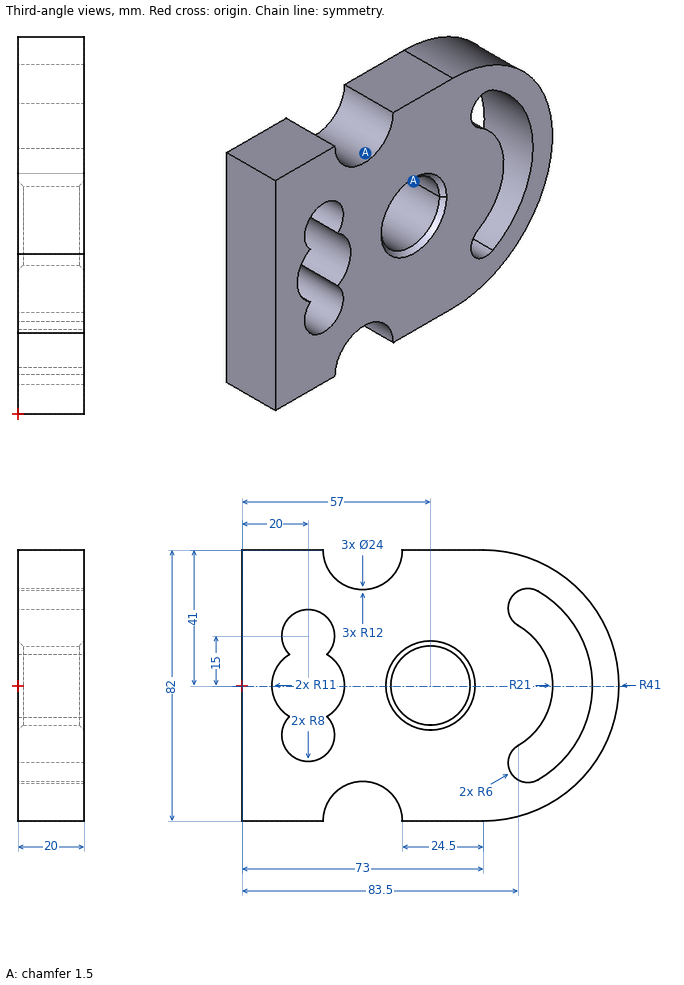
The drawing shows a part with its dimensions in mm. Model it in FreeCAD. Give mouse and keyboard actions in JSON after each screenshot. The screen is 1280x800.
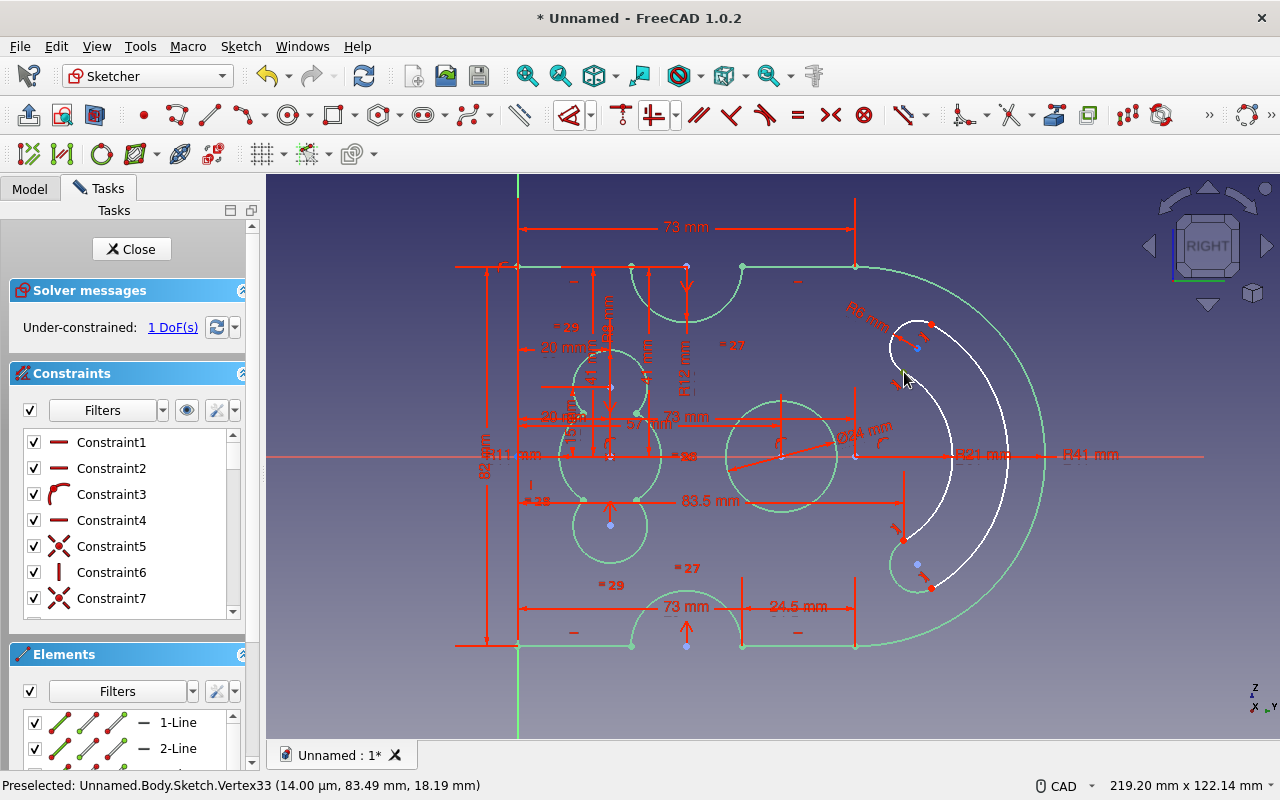
{"action": "key", "text": "l"}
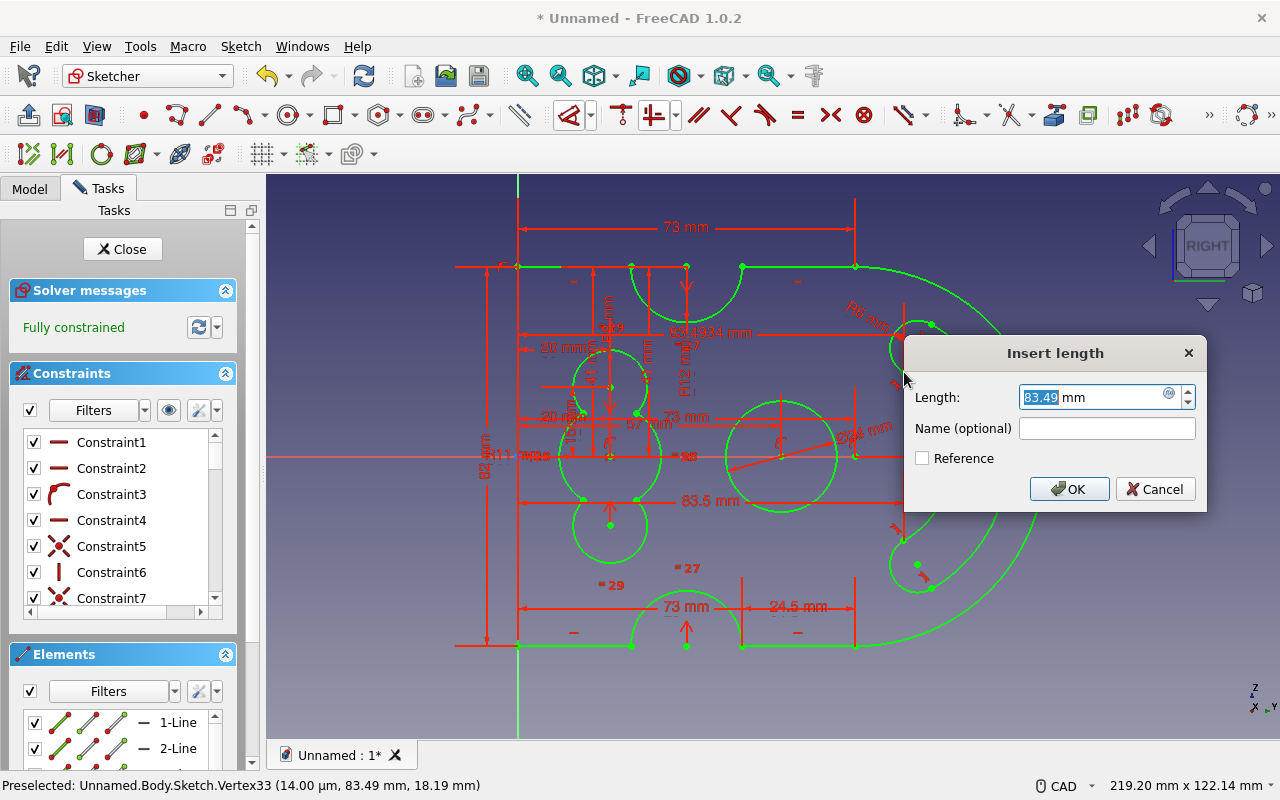
{"action": "type", "text": "83.5"}
{"action": "key", "text": "Return"}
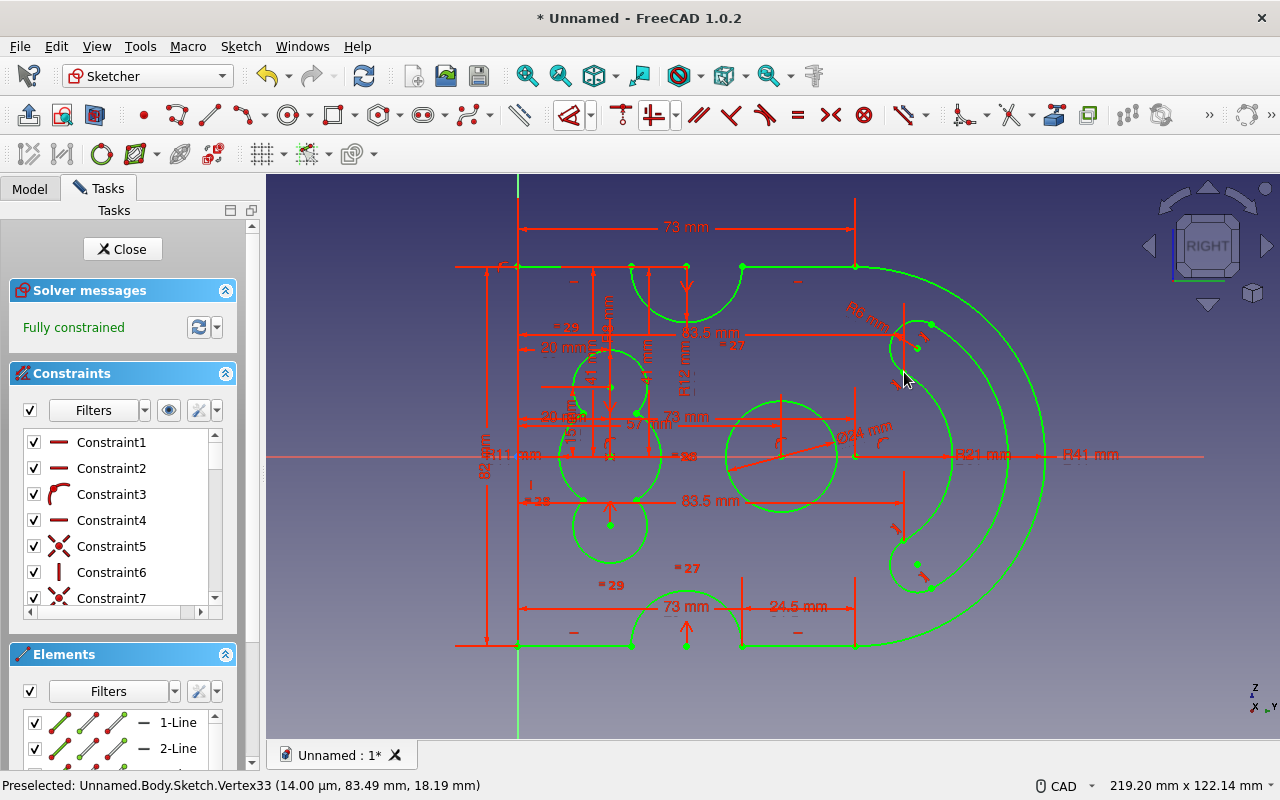
{"action": "left_click", "coordinate": [123, 249]}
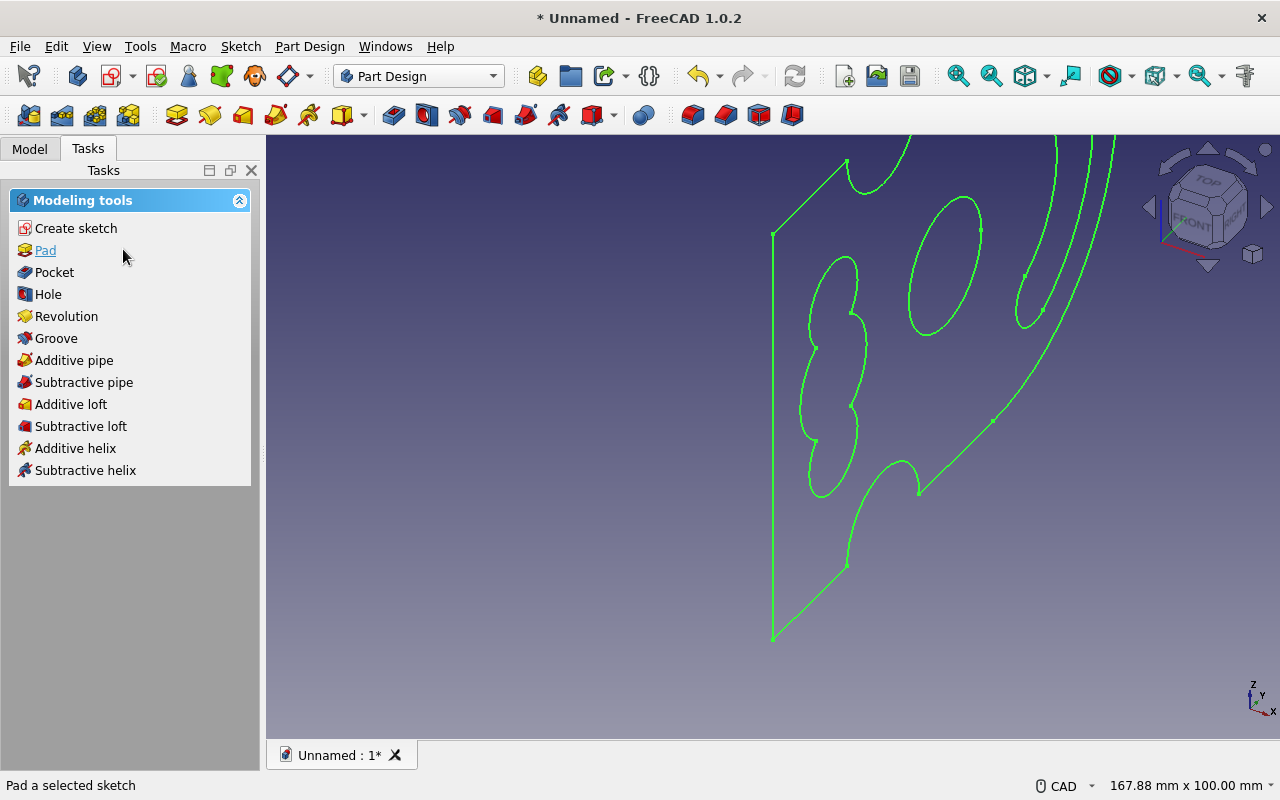
{"action": "left_click", "coordinate": [177, 116]}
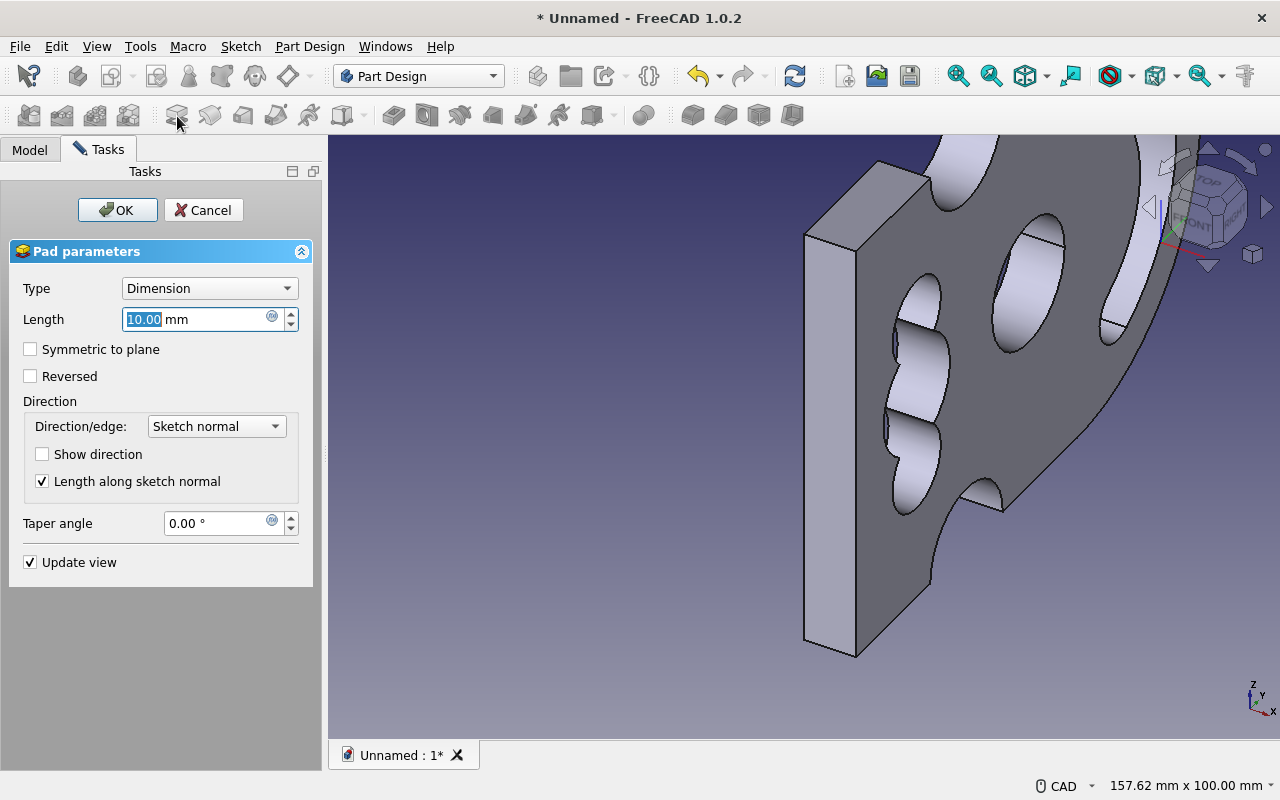
{"action": "type", "text": "20"}
{"action": "key", "text": "Tab"}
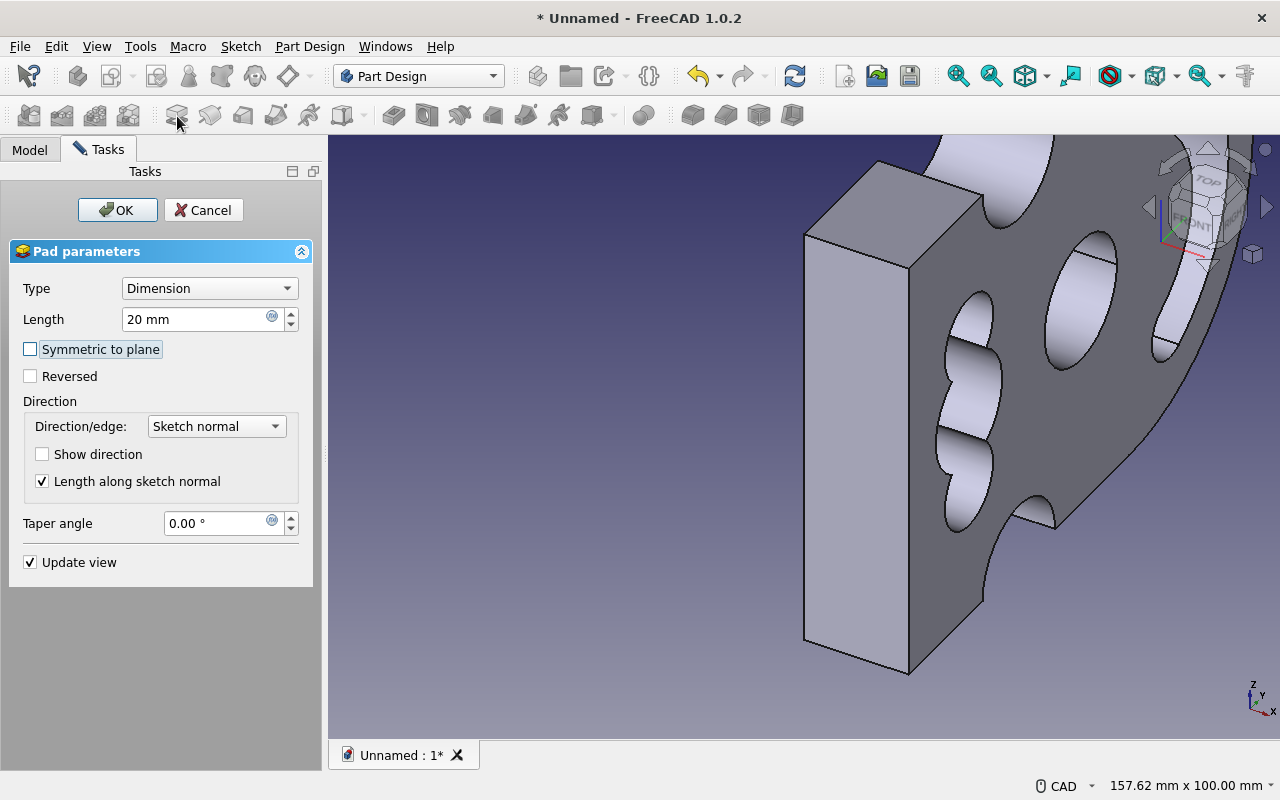
{"action": "left_click", "coordinate": [118, 210]}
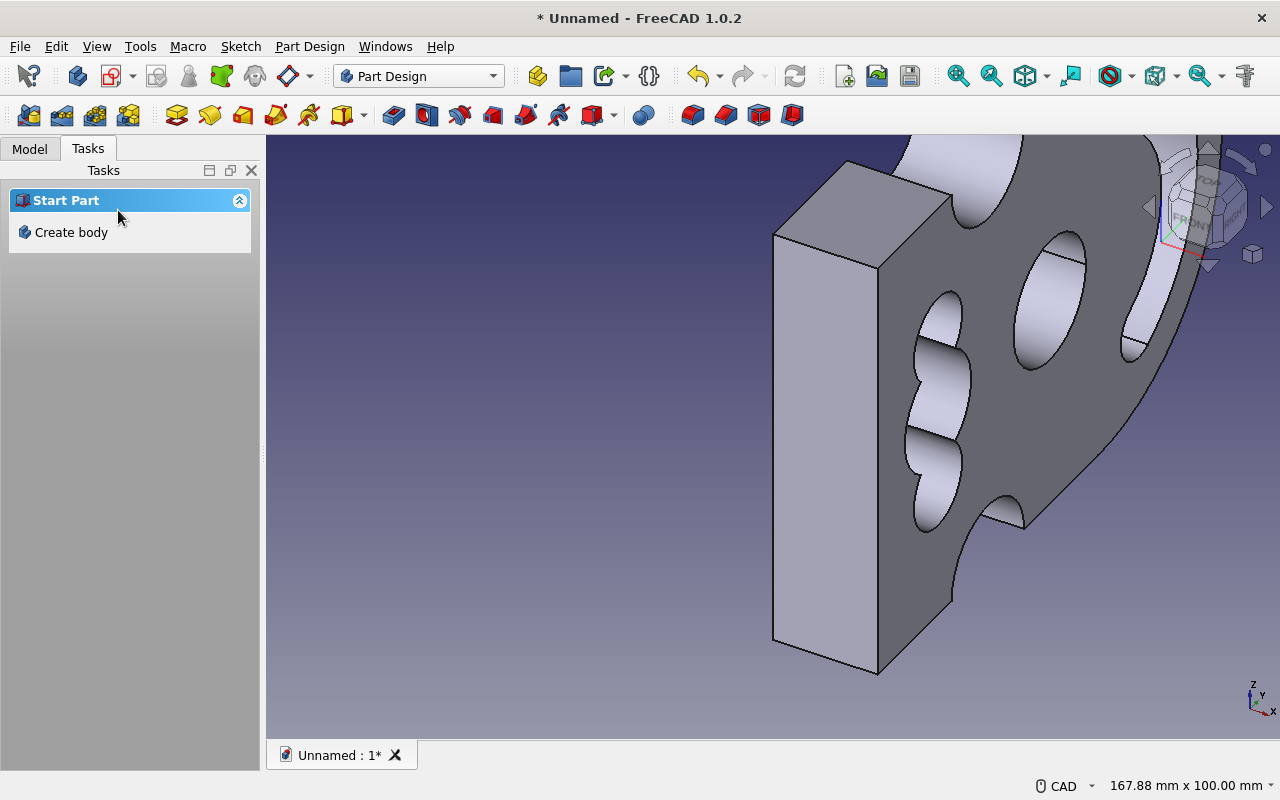
{"action": "left_click", "coordinate": [959, 76]}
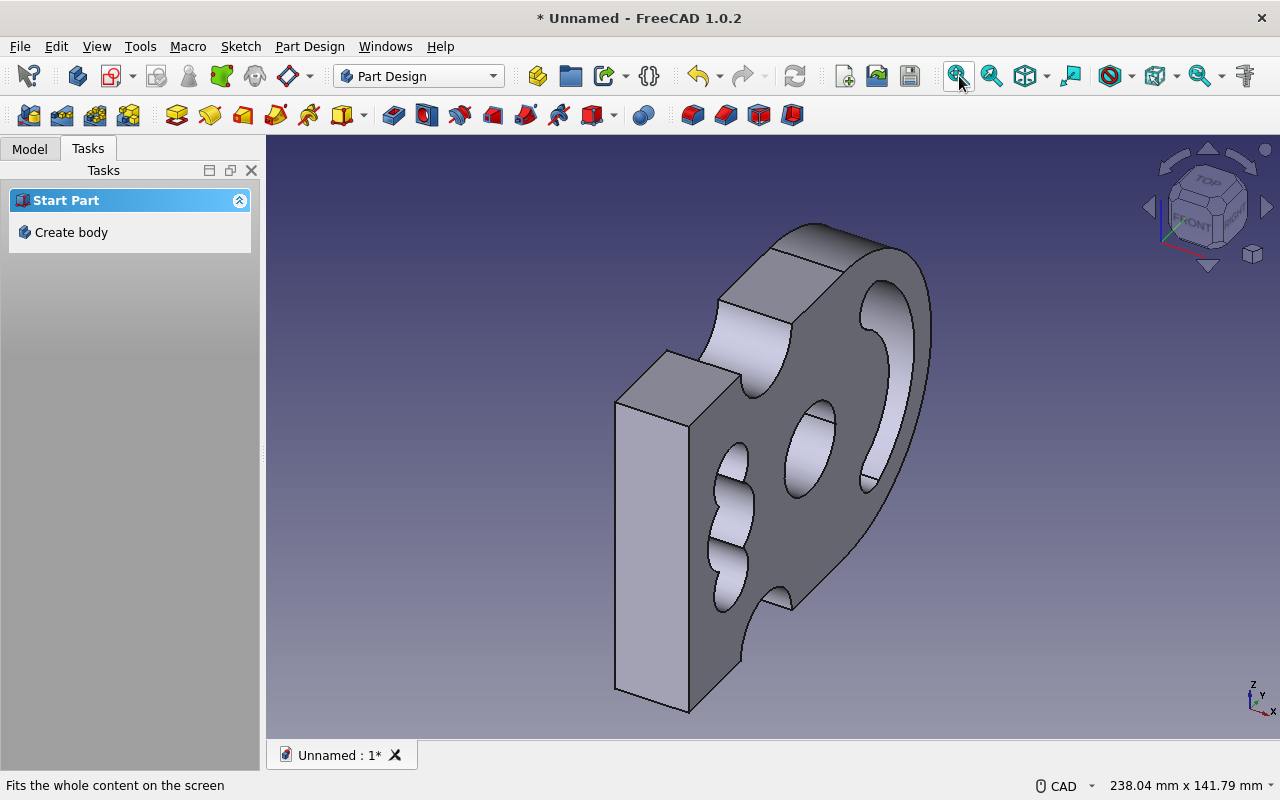
{"action": "left_click", "coordinate": [802, 496]}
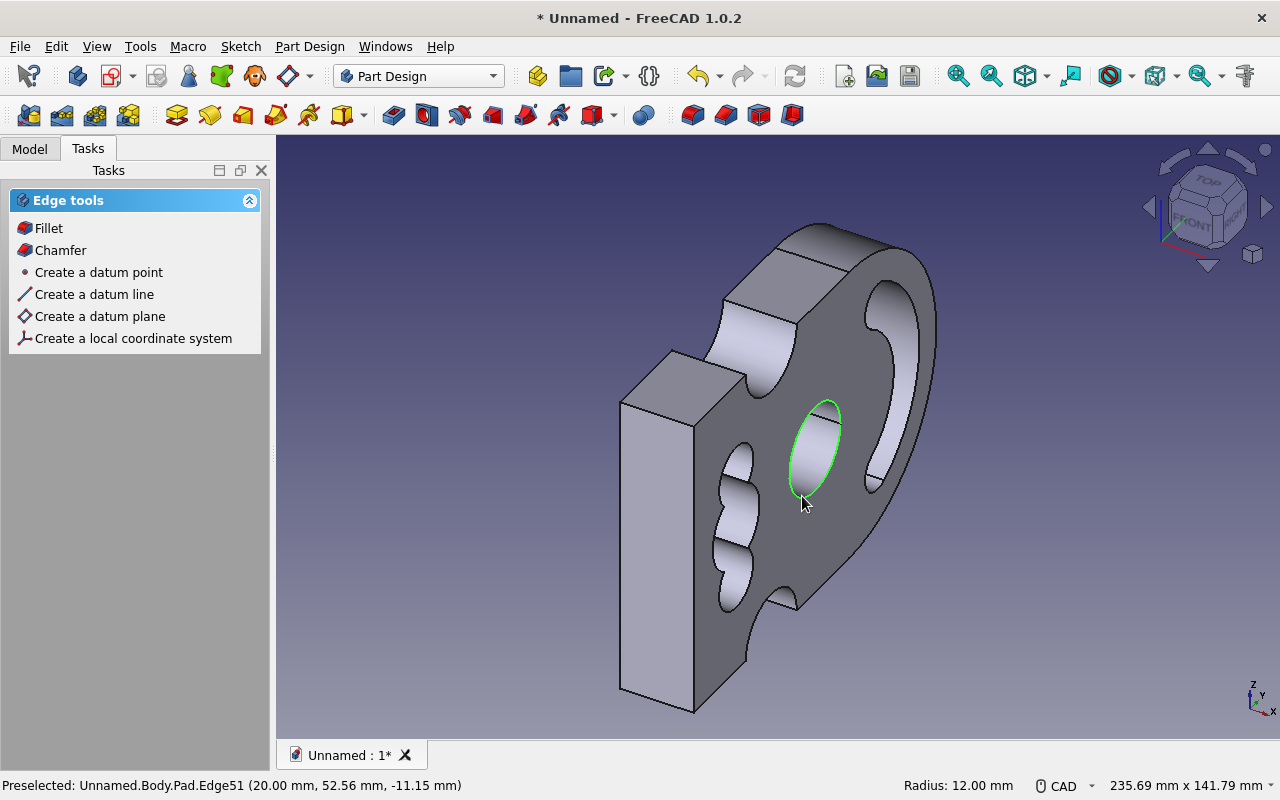
{"action": "key", "text": "0"}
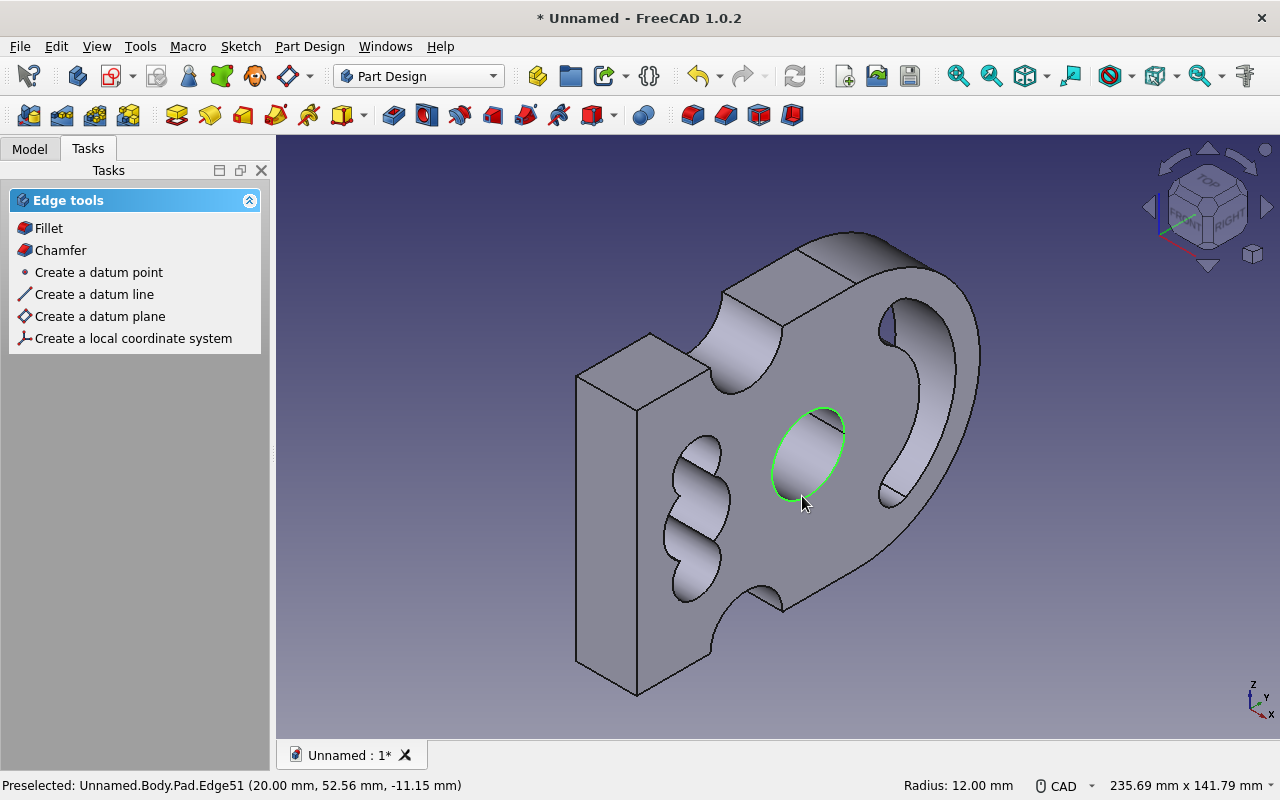
{"action": "key", "text": "2"}